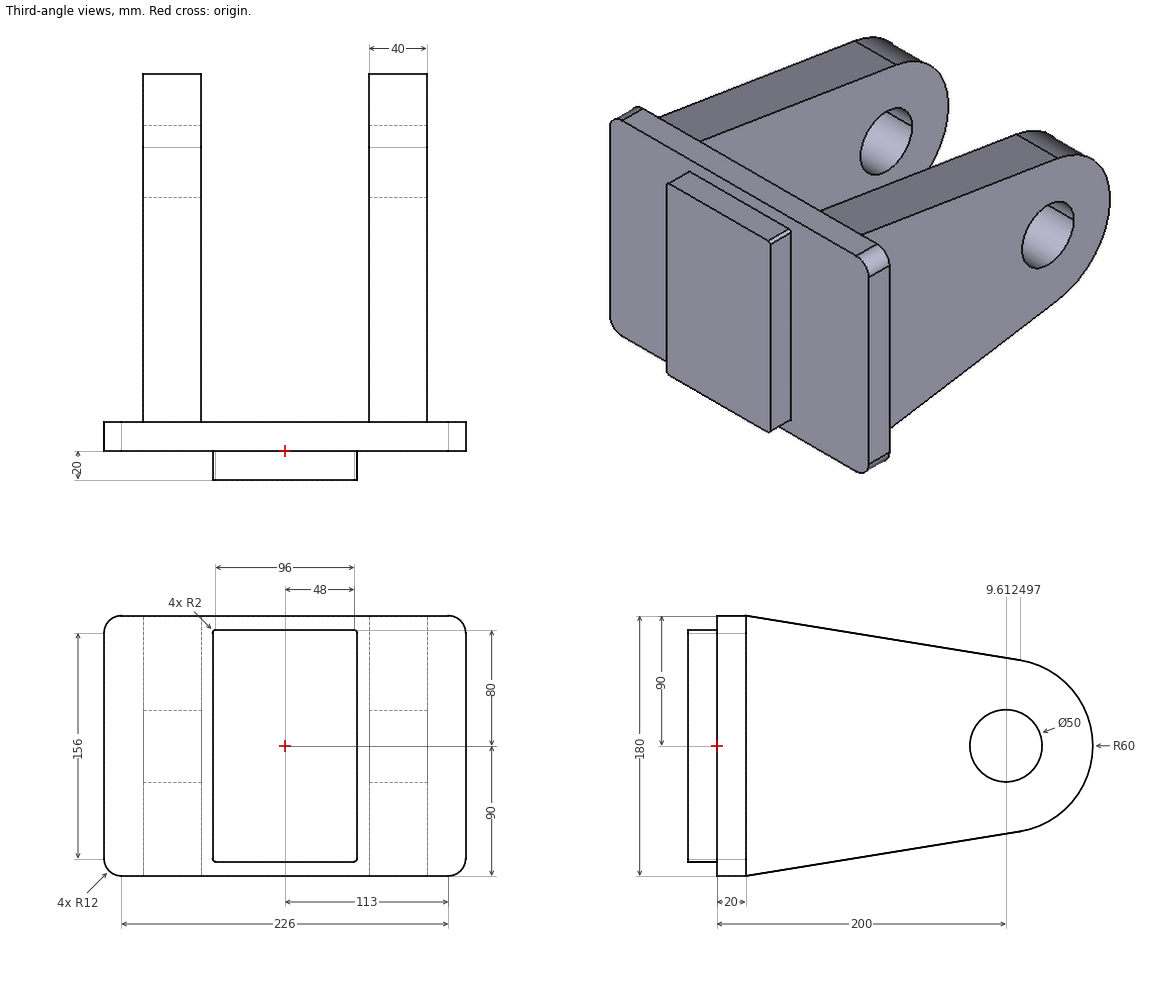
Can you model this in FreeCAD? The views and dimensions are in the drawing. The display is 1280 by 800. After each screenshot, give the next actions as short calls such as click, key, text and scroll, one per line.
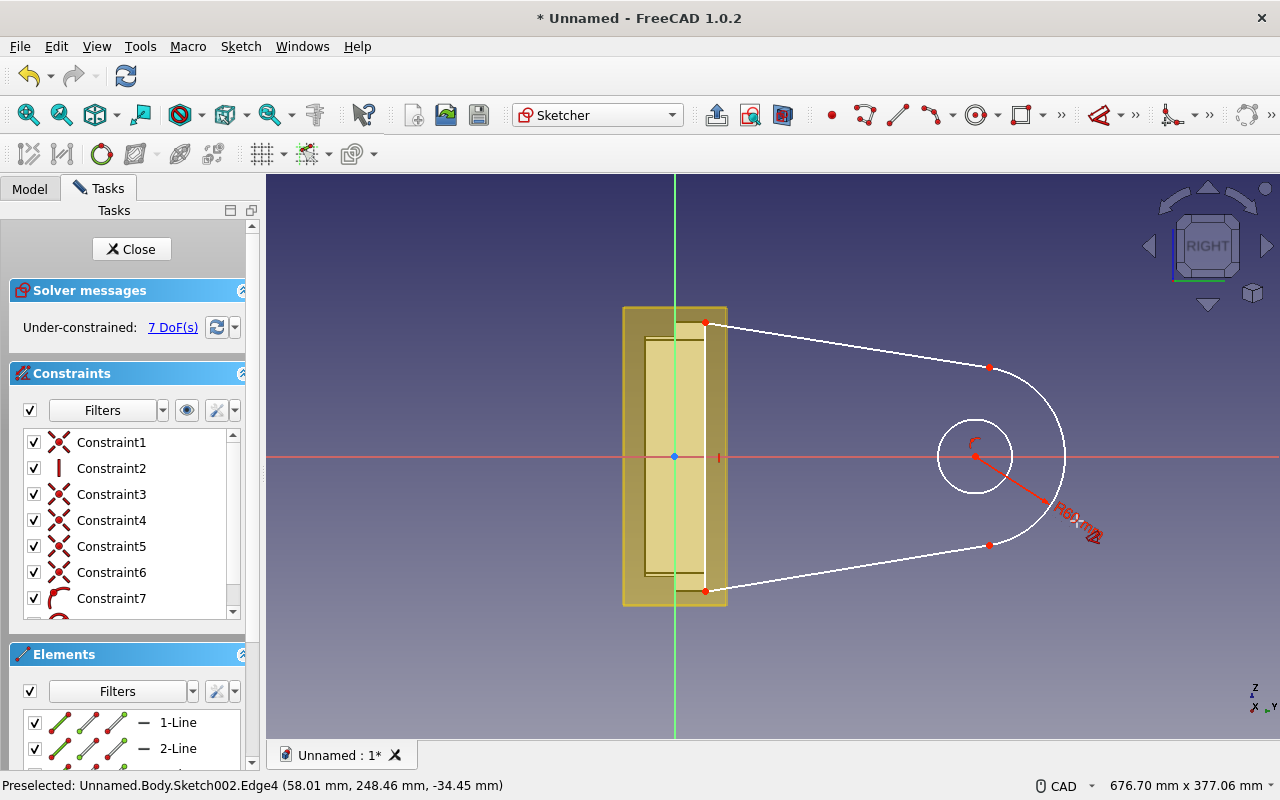
click(1001, 430)
click(1023, 407)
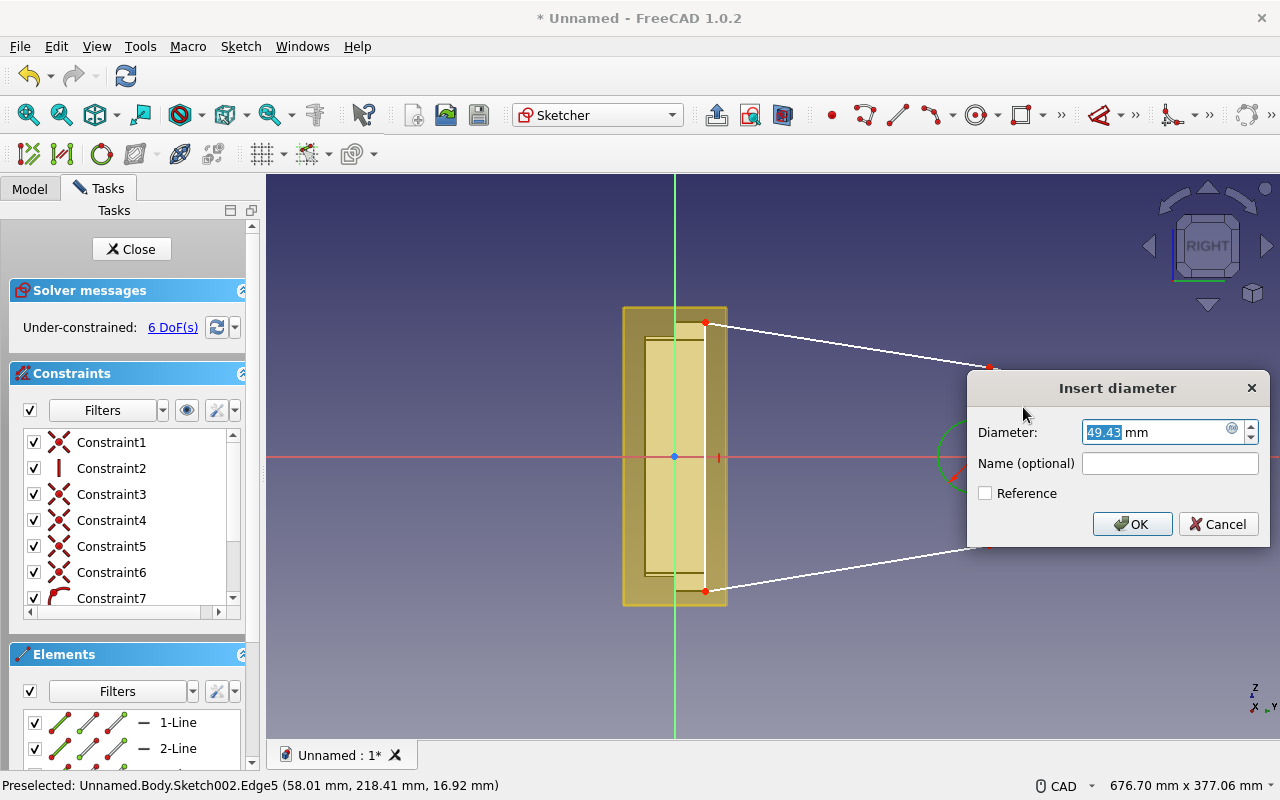
text(50)
key(Return)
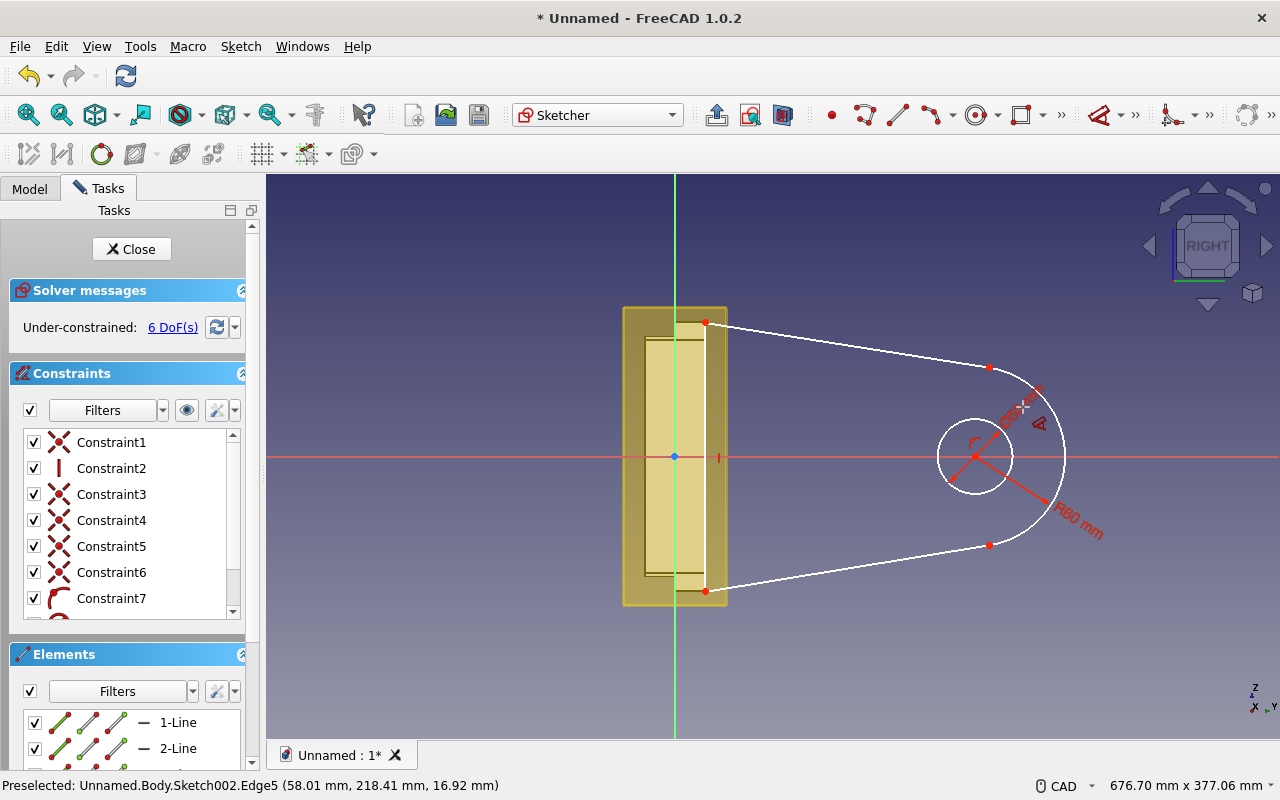
click(705, 404)
click(739, 396)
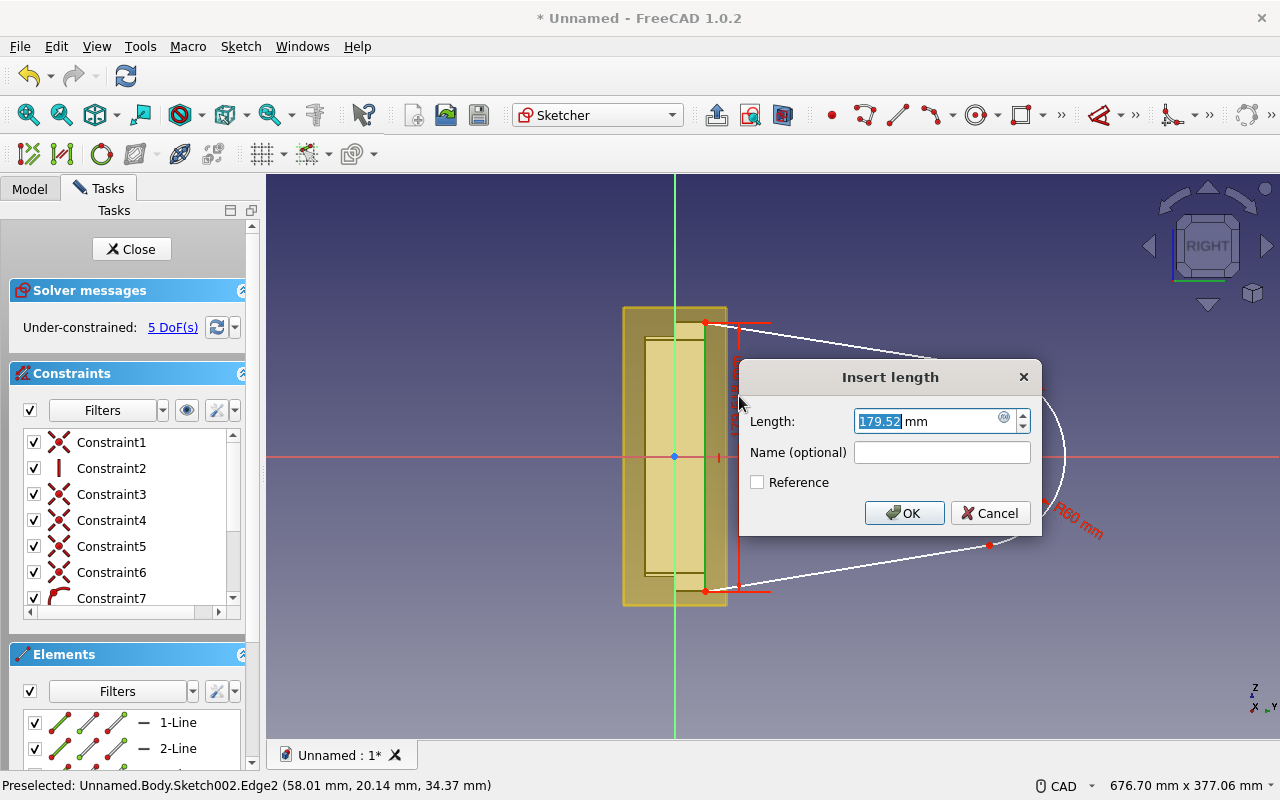
text(180)
key(Return)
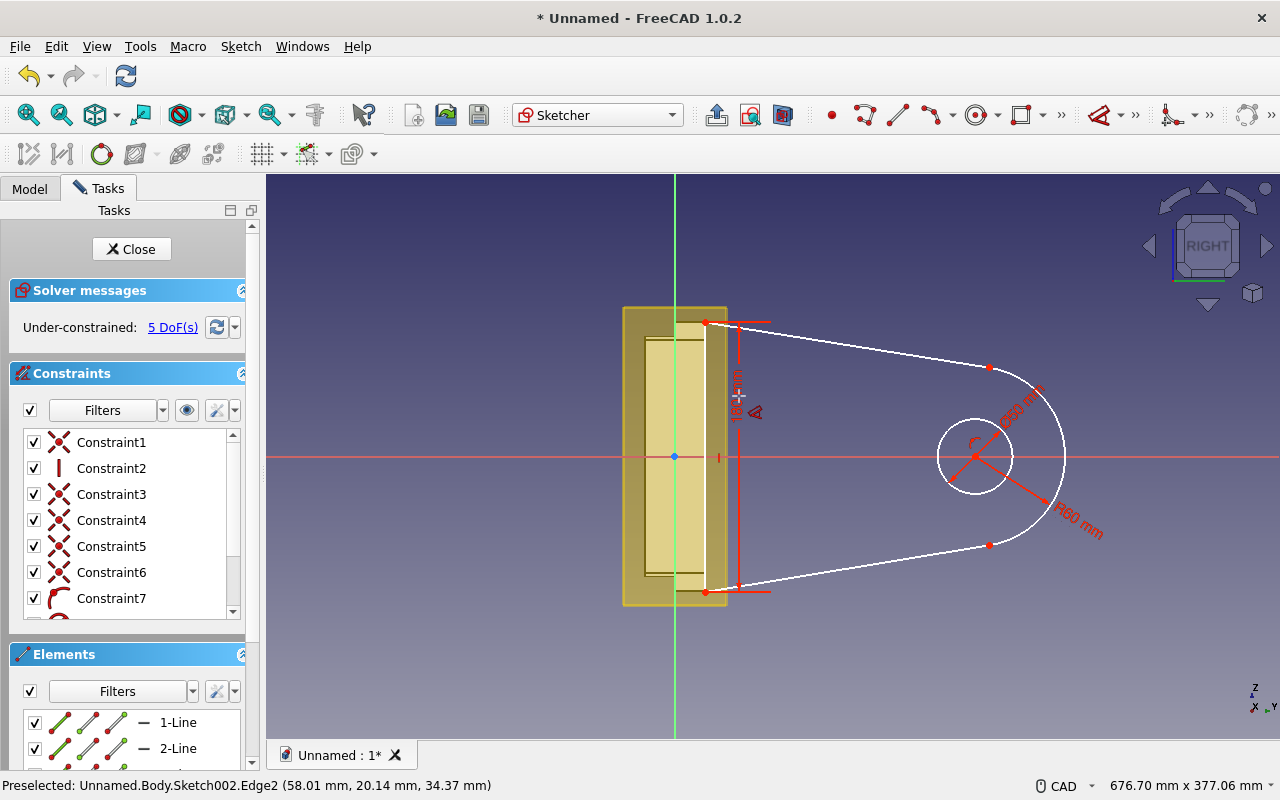
scroll(705, 322, up, 2)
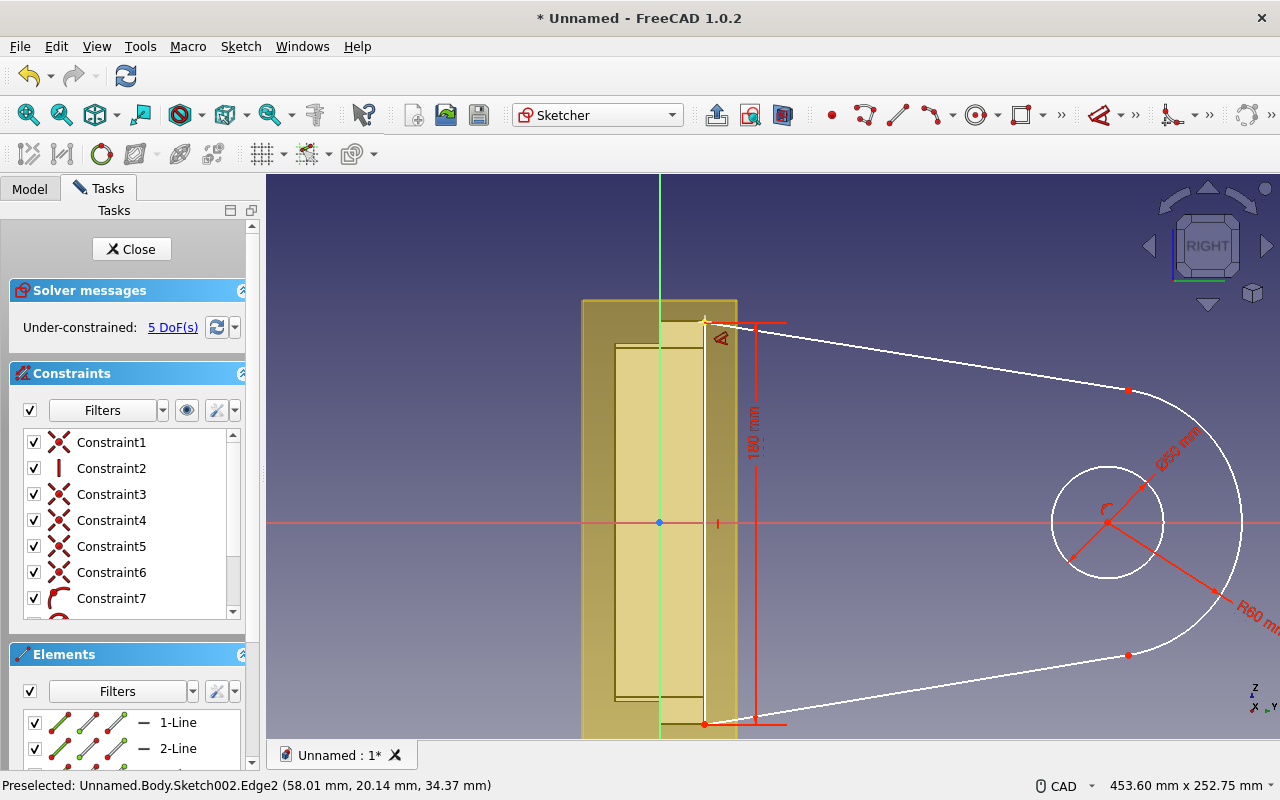
click(705, 323)
click(682, 289)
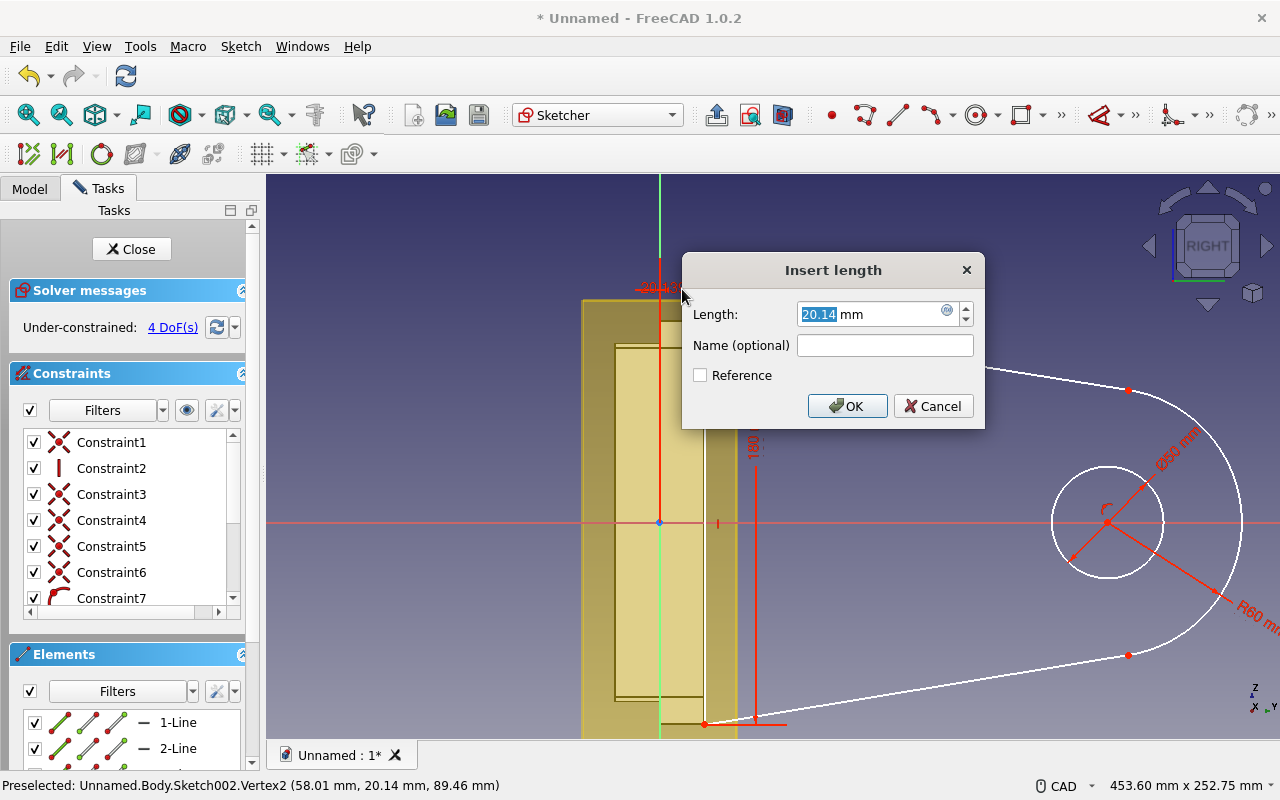
text(20)
key(Return)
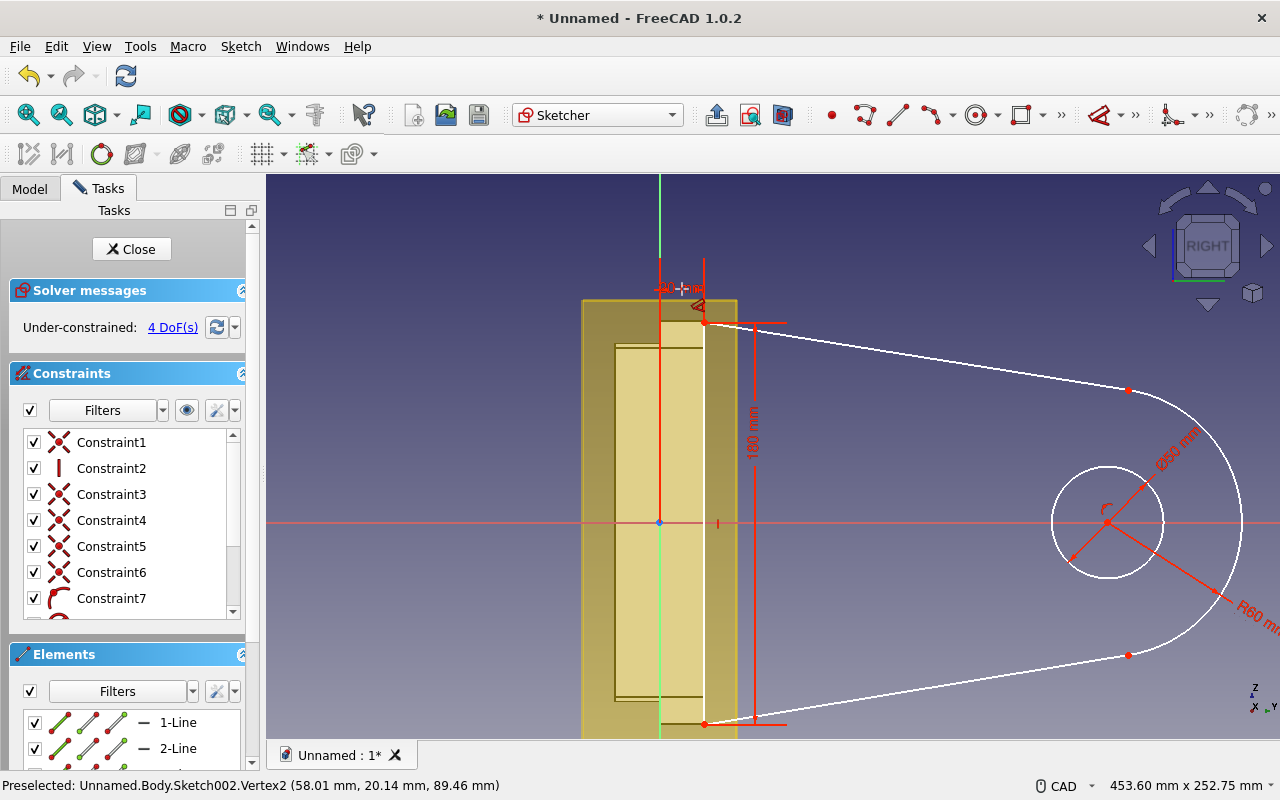
click(704, 323)
click(626, 423)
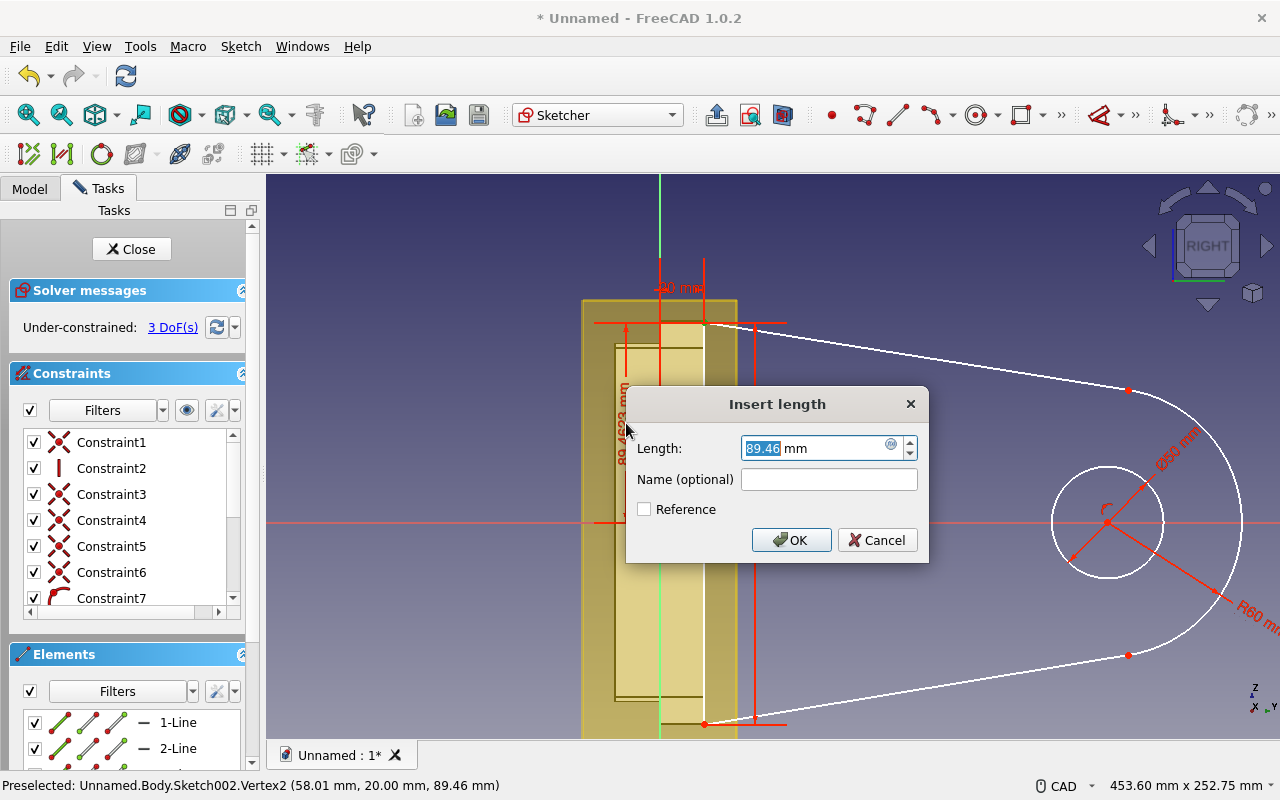
text(90)
key(Return)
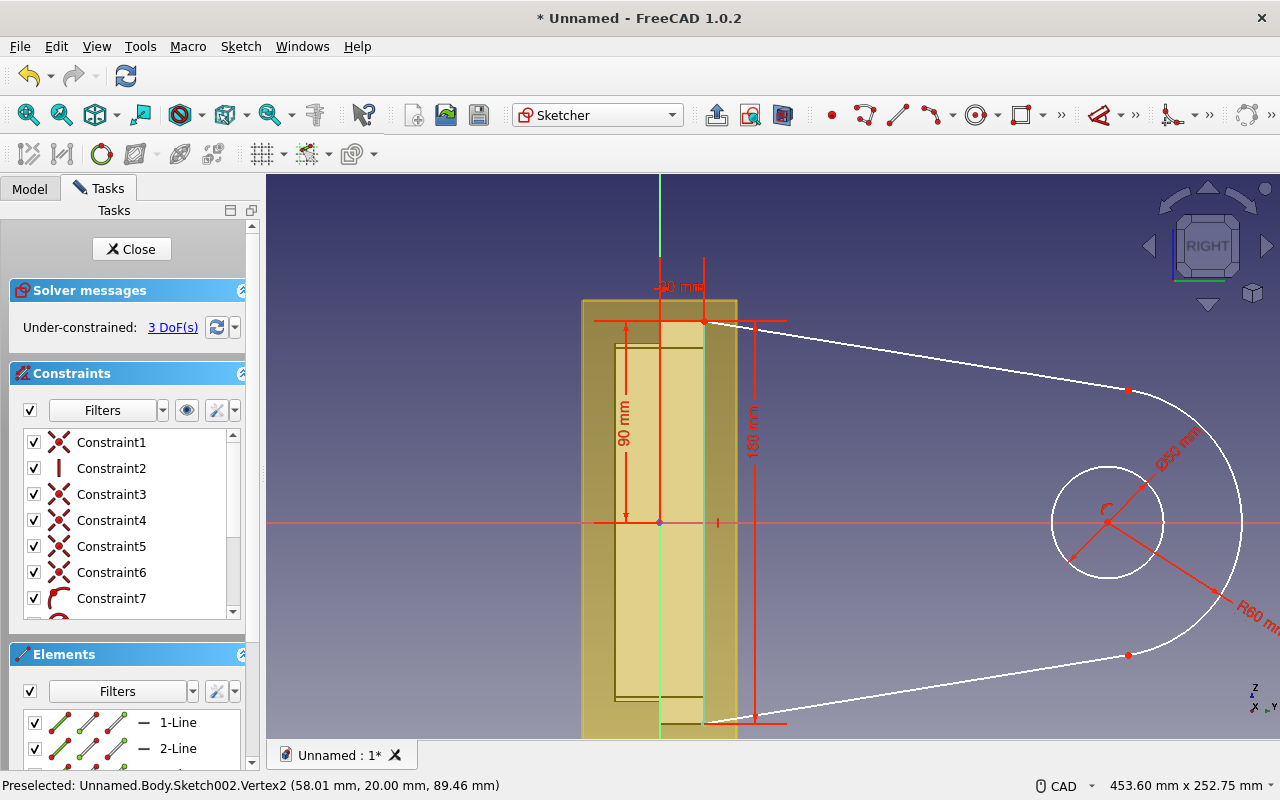
click(1108, 523)
click(884, 557)